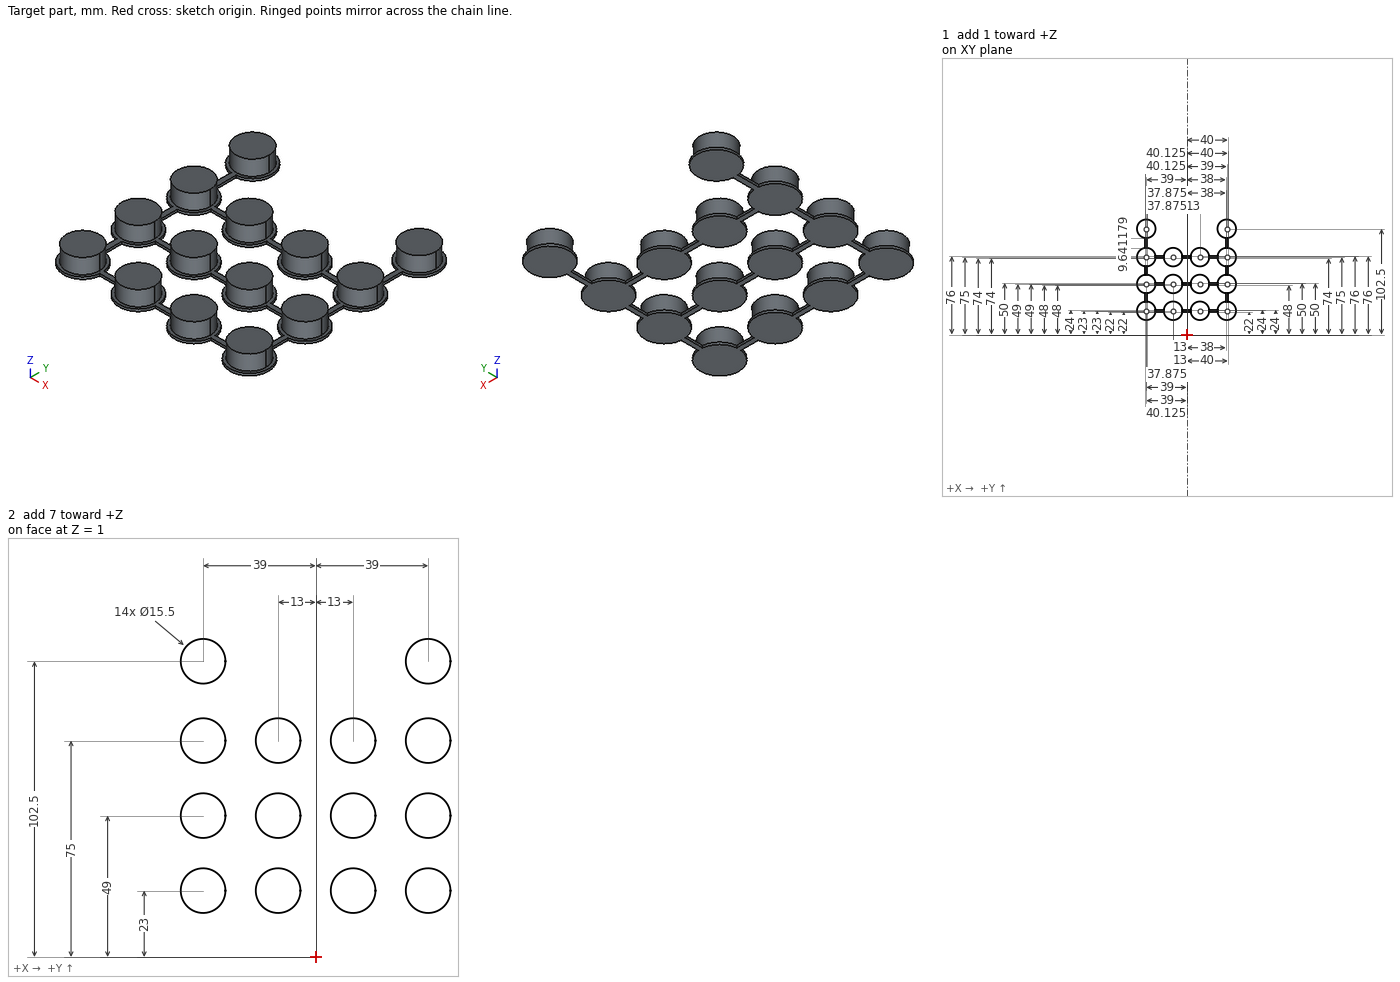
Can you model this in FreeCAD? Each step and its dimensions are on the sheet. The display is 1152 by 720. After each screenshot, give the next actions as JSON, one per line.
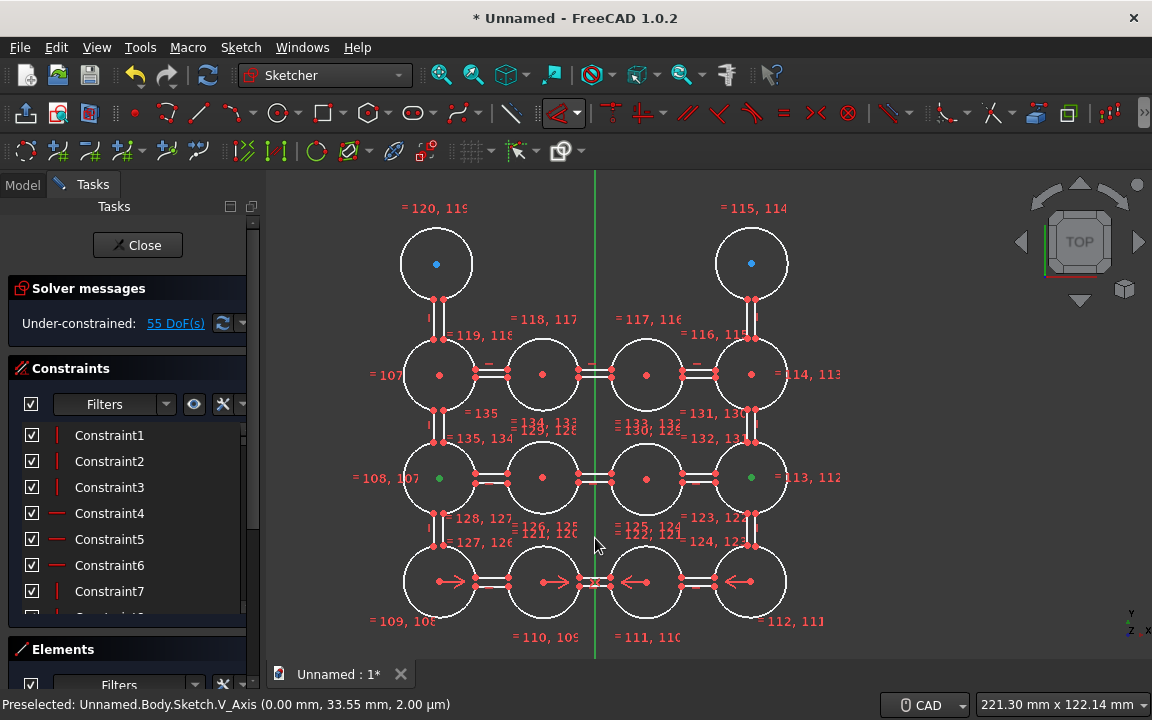
{"action": "left_click", "coordinate": [816, 114]}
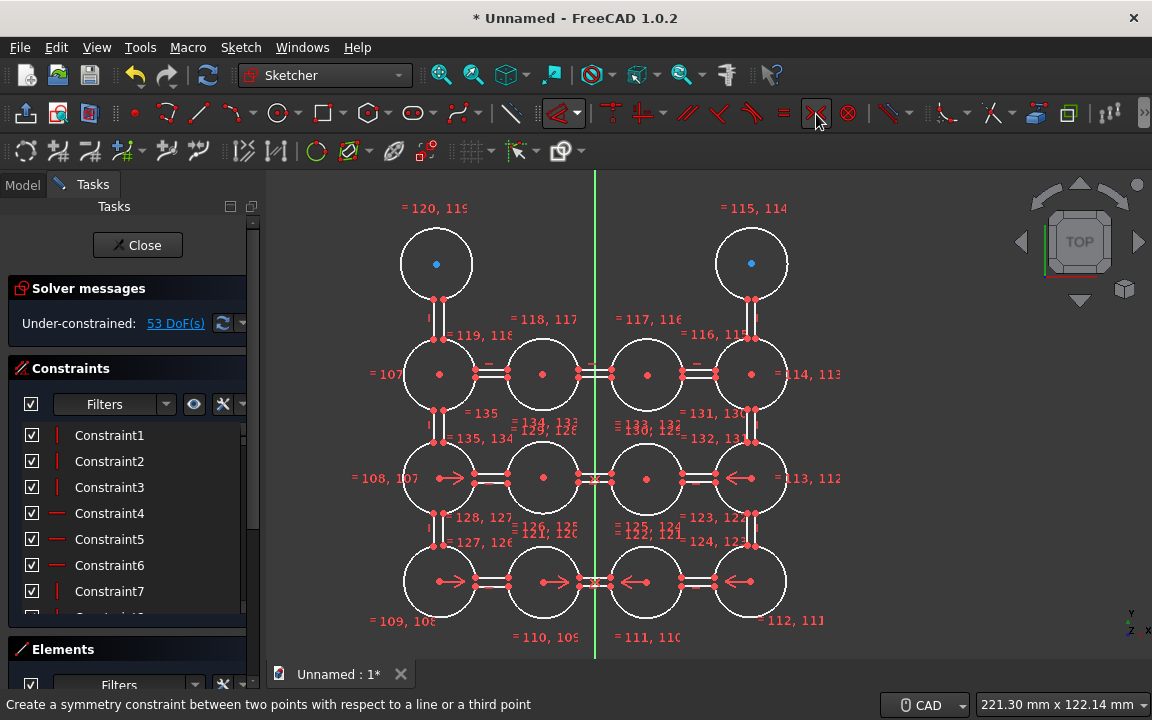
{"action": "left_click", "coordinate": [440, 375]}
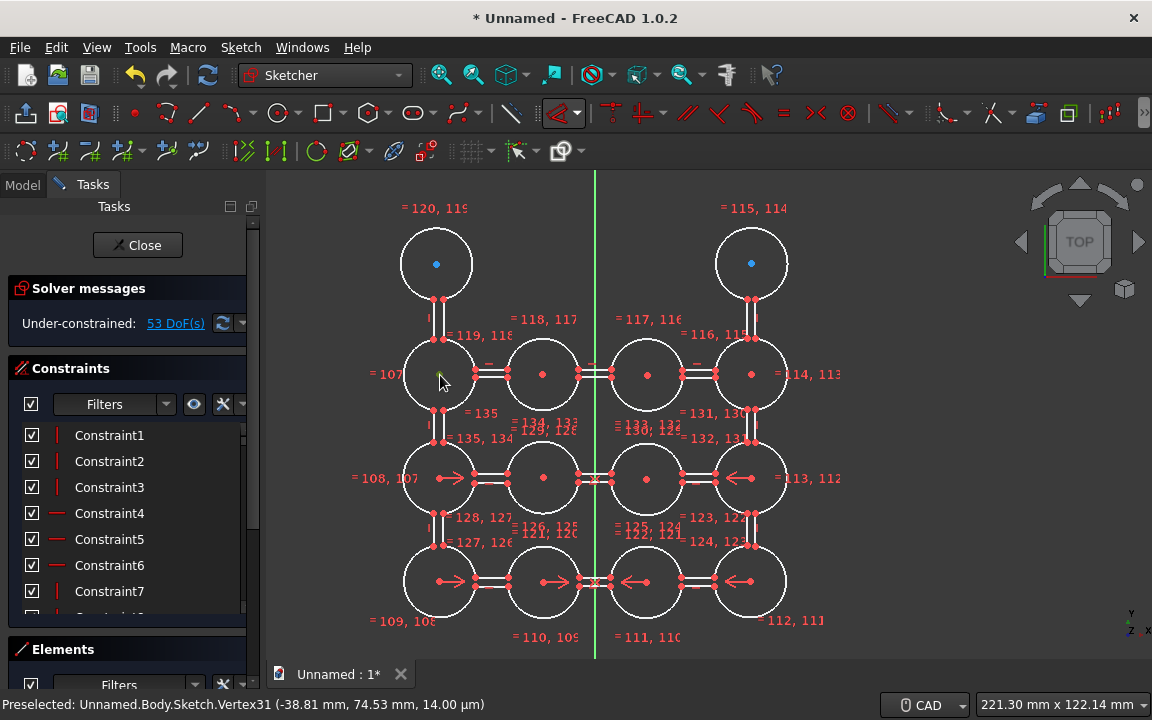
{"action": "left_click", "coordinate": [751, 374]}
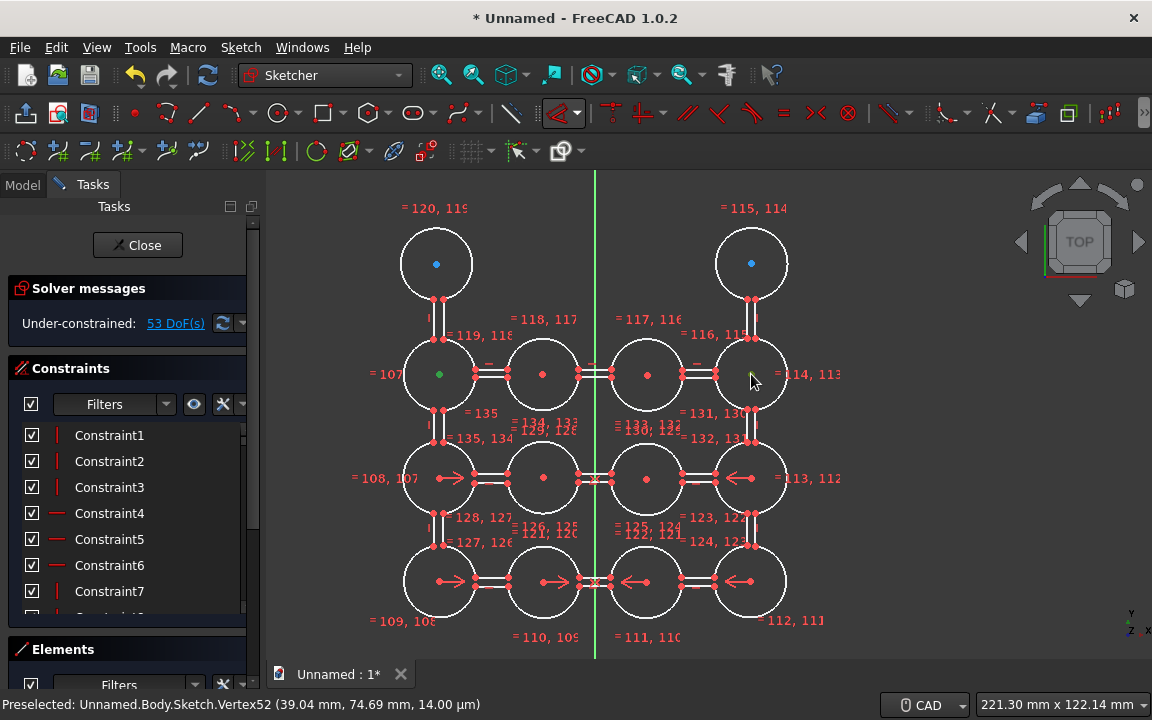
{"action": "left_click", "coordinate": [595, 538]}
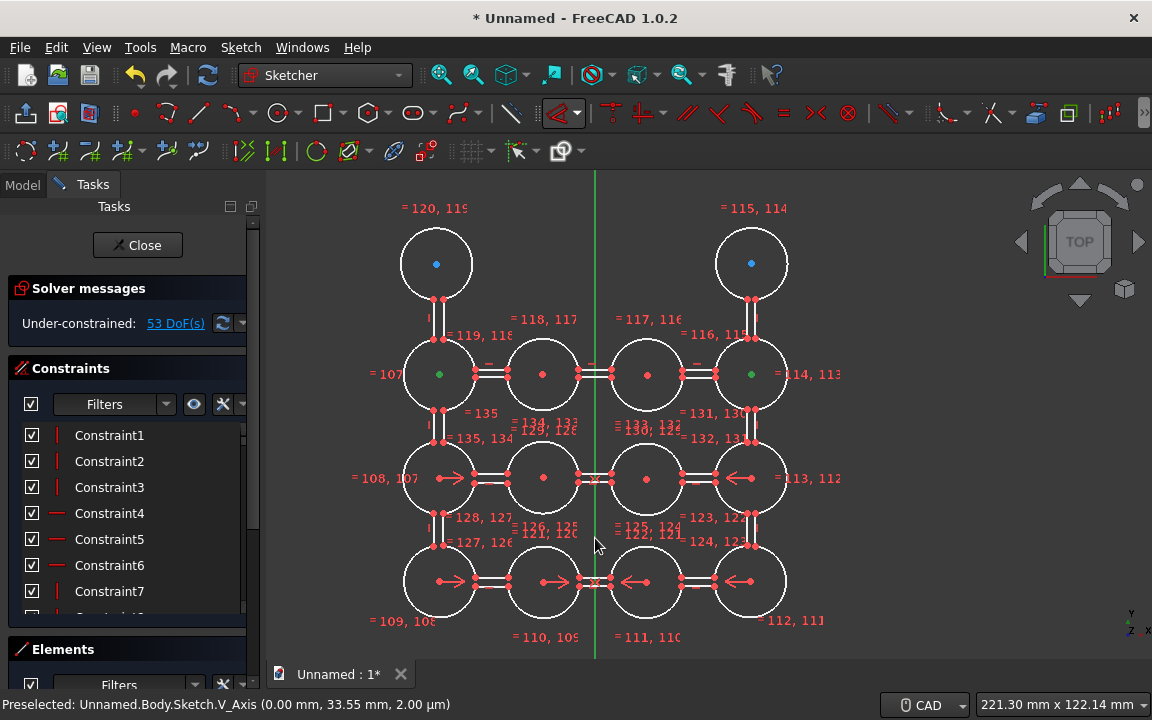
{"action": "left_click", "coordinate": [816, 114]}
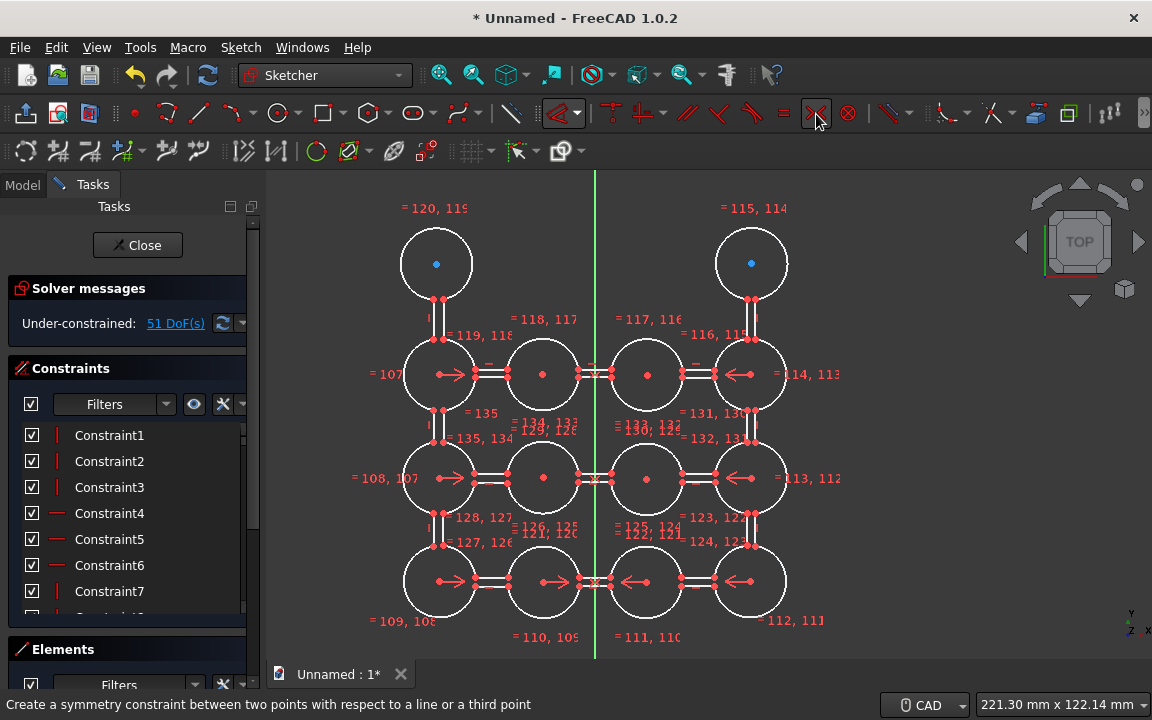
{"action": "left_click", "coordinate": [647, 375]}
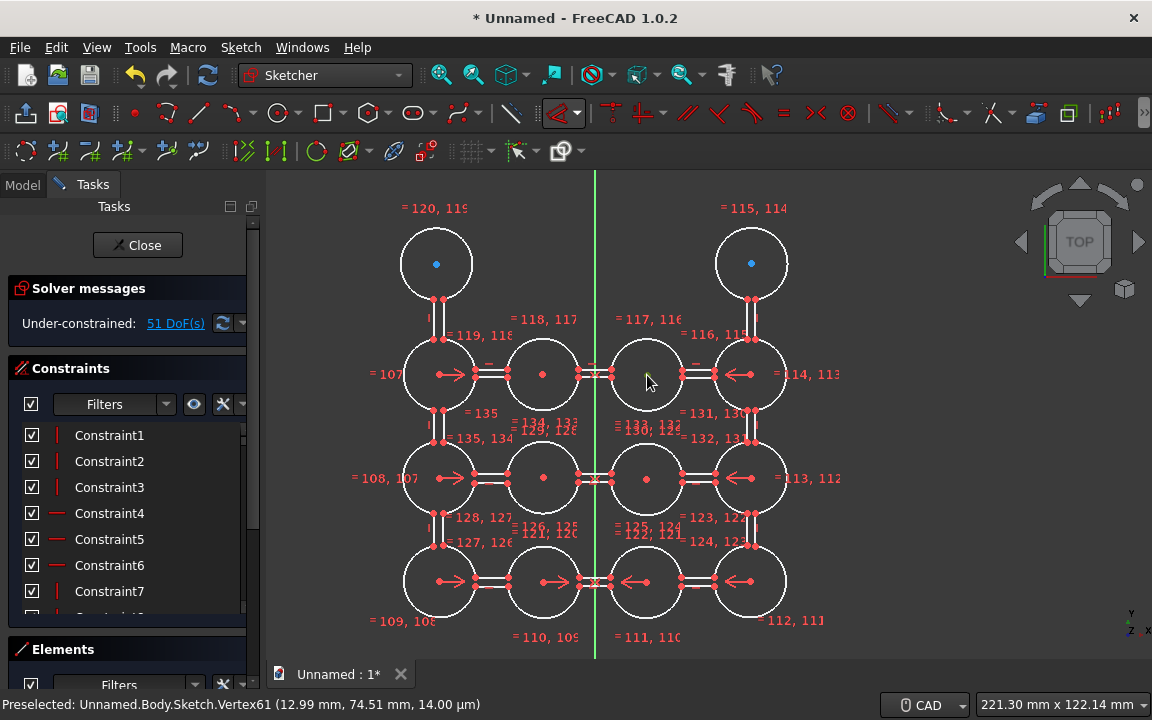
{"action": "left_click", "coordinate": [543, 375]}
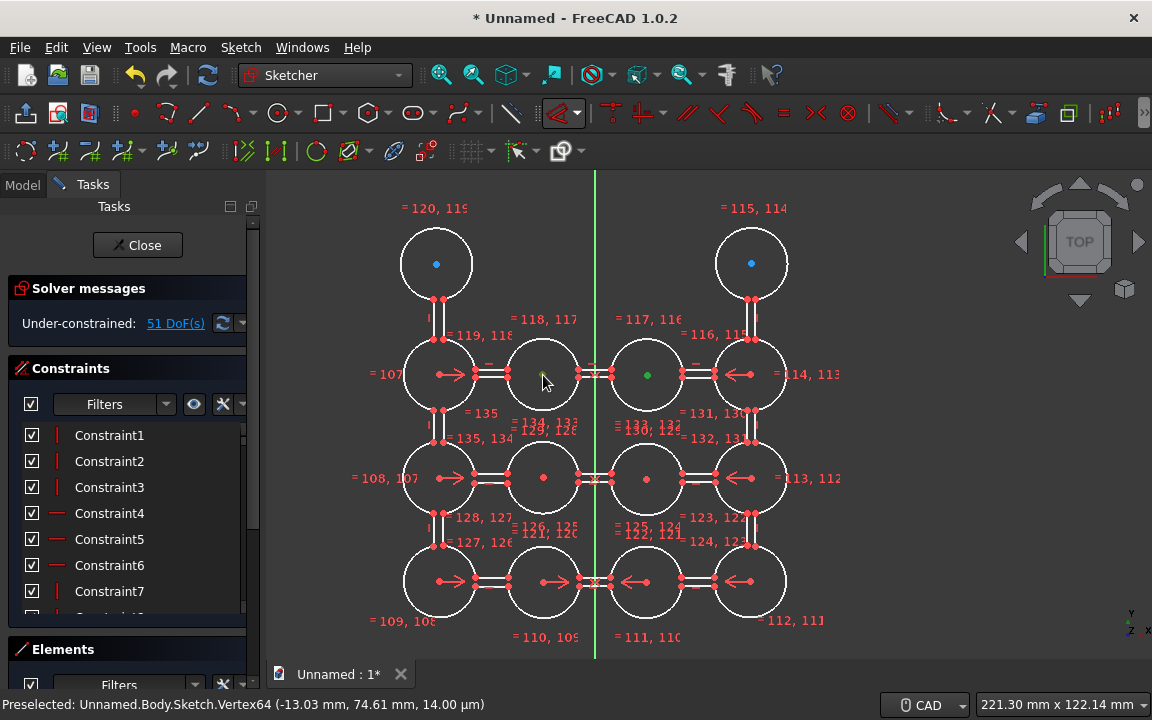
{"action": "left_click", "coordinate": [595, 538]}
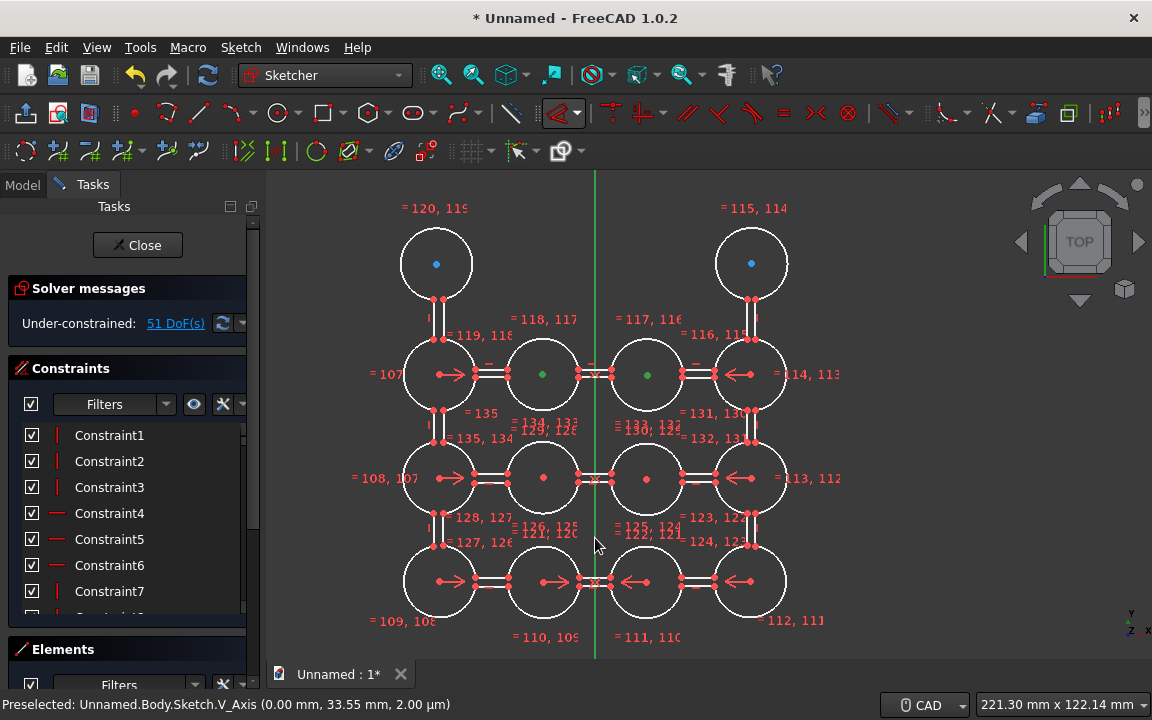
{"action": "left_click", "coordinate": [816, 114]}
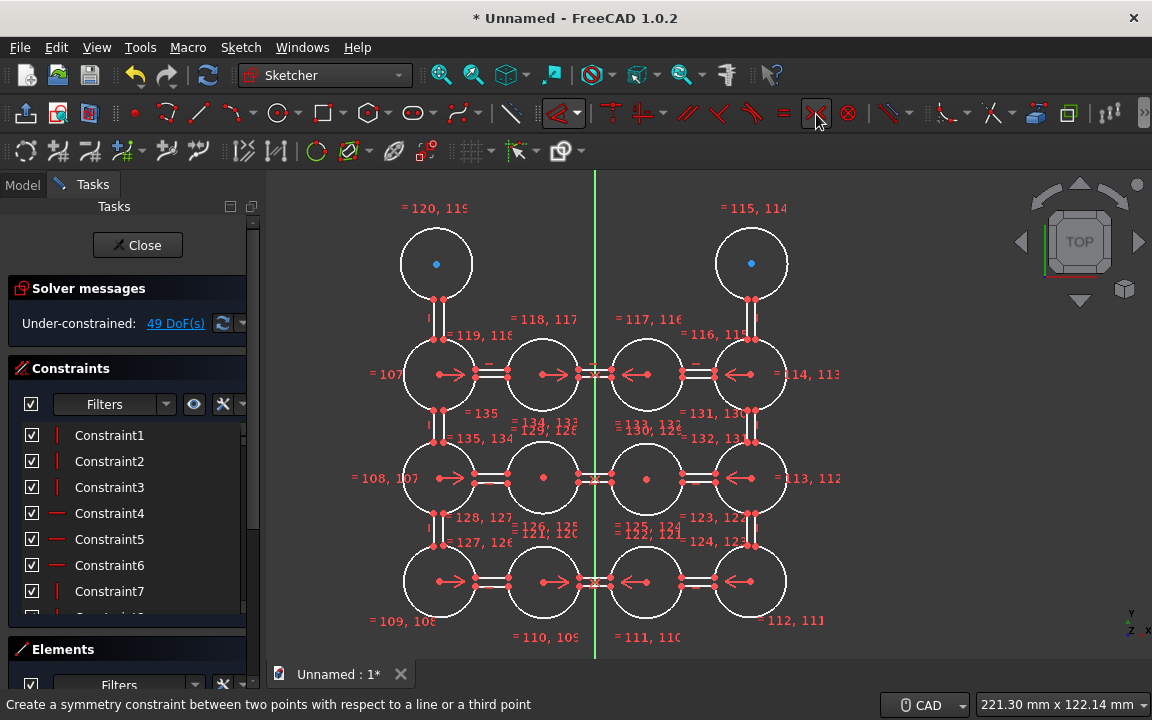
{"action": "left_click", "coordinate": [752, 264]}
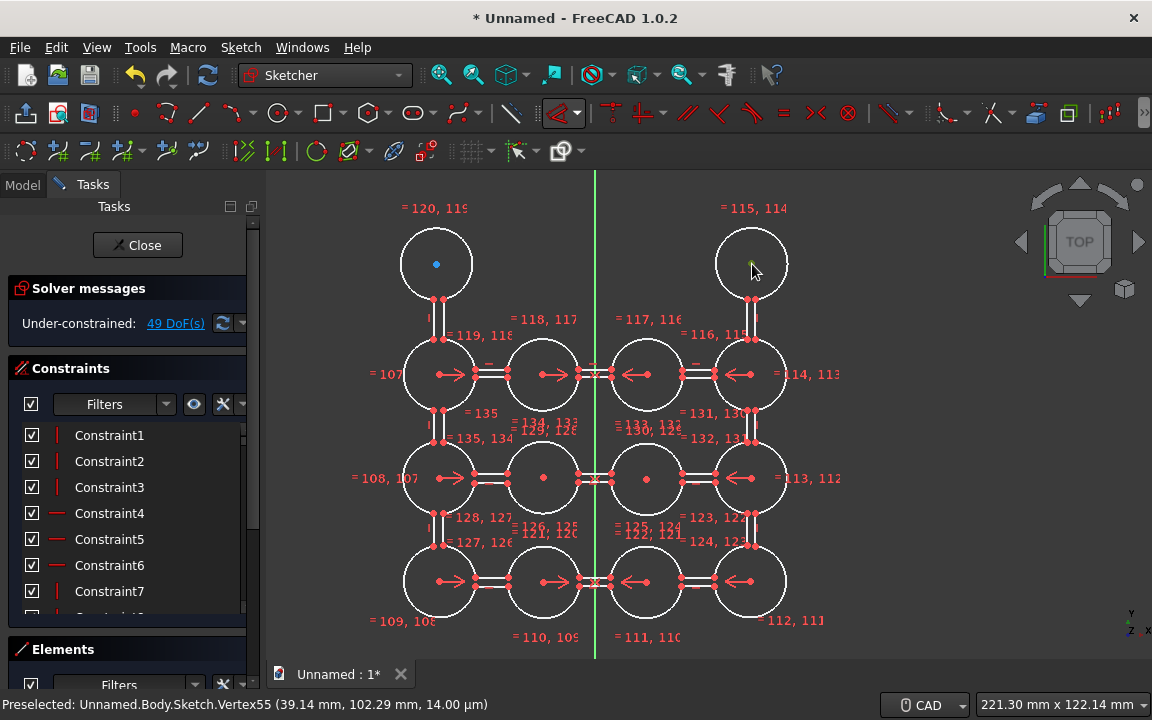
{"action": "left_click", "coordinate": [437, 264]}